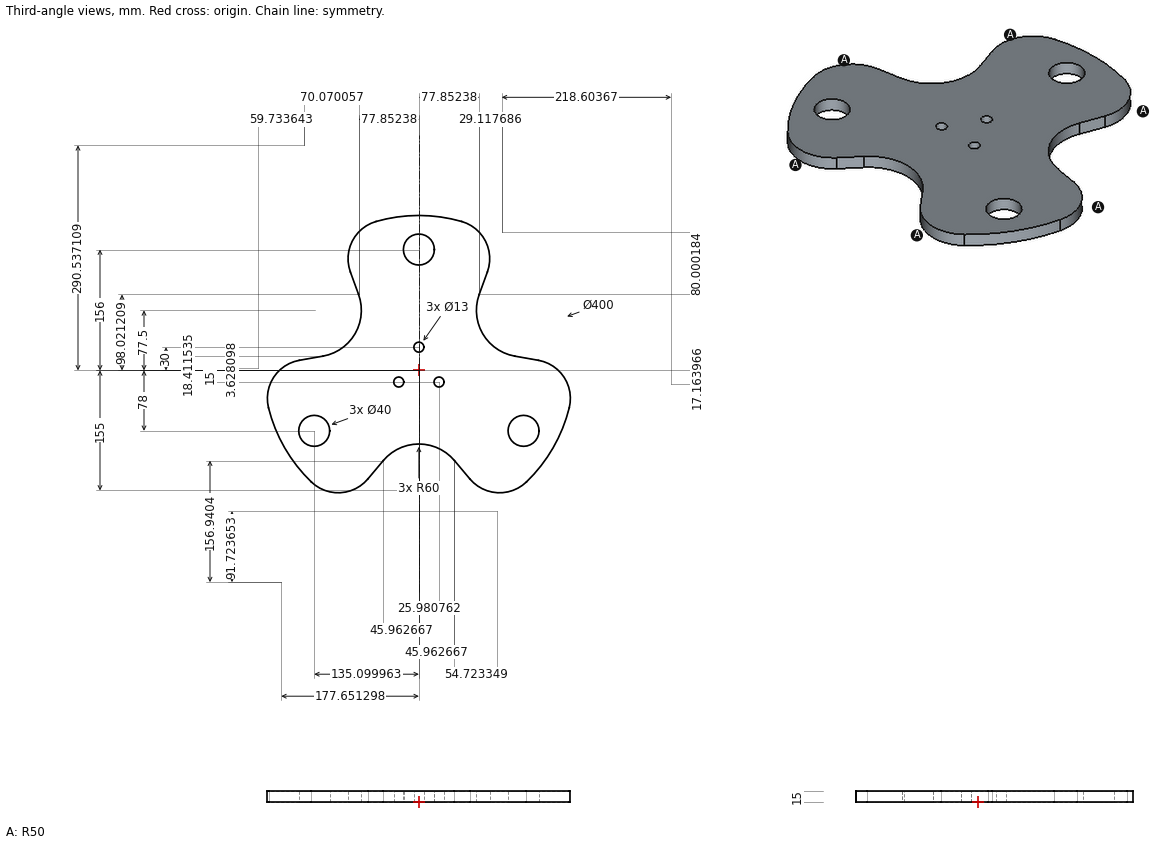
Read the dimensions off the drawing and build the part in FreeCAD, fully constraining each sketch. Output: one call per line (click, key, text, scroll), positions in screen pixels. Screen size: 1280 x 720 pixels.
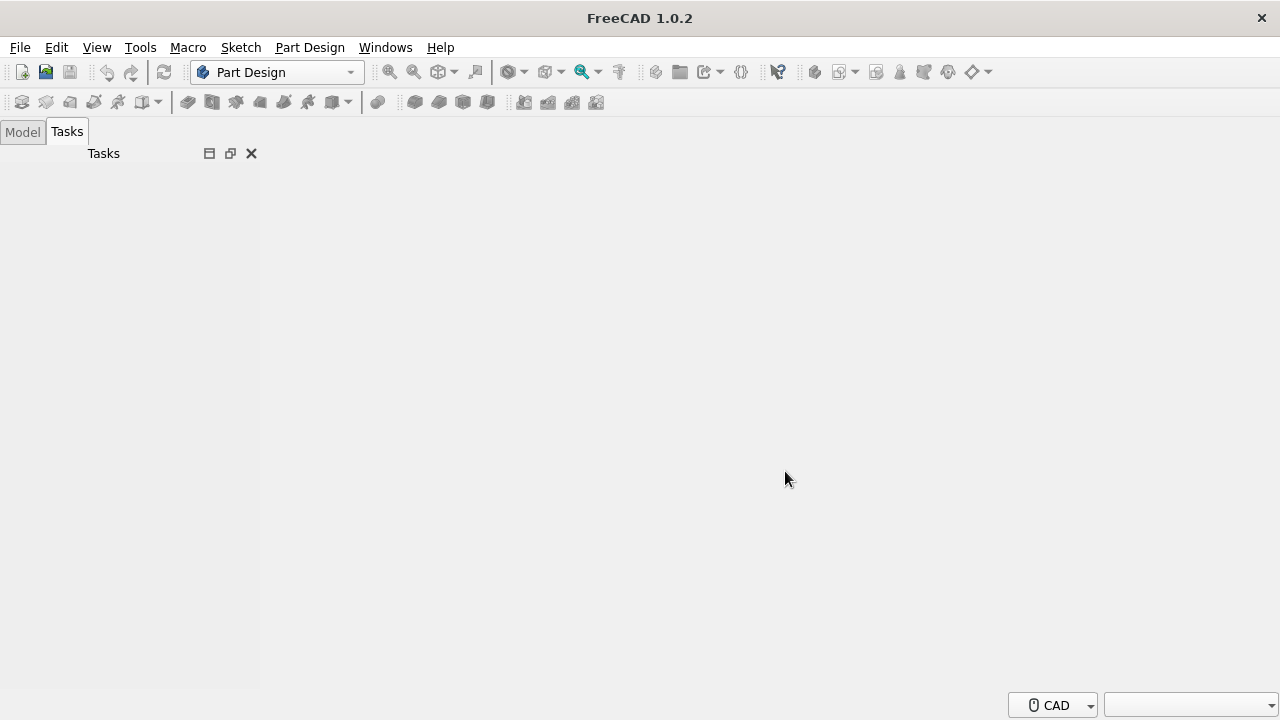
click(22, 72)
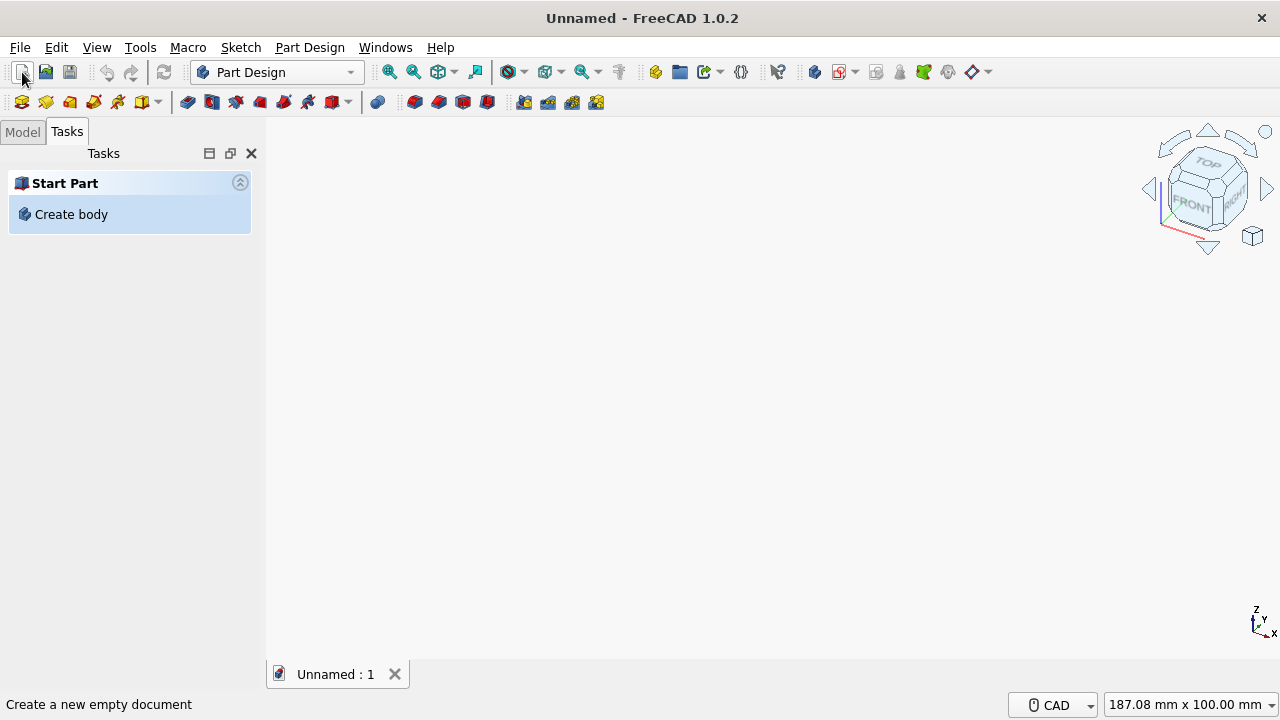
click(840, 72)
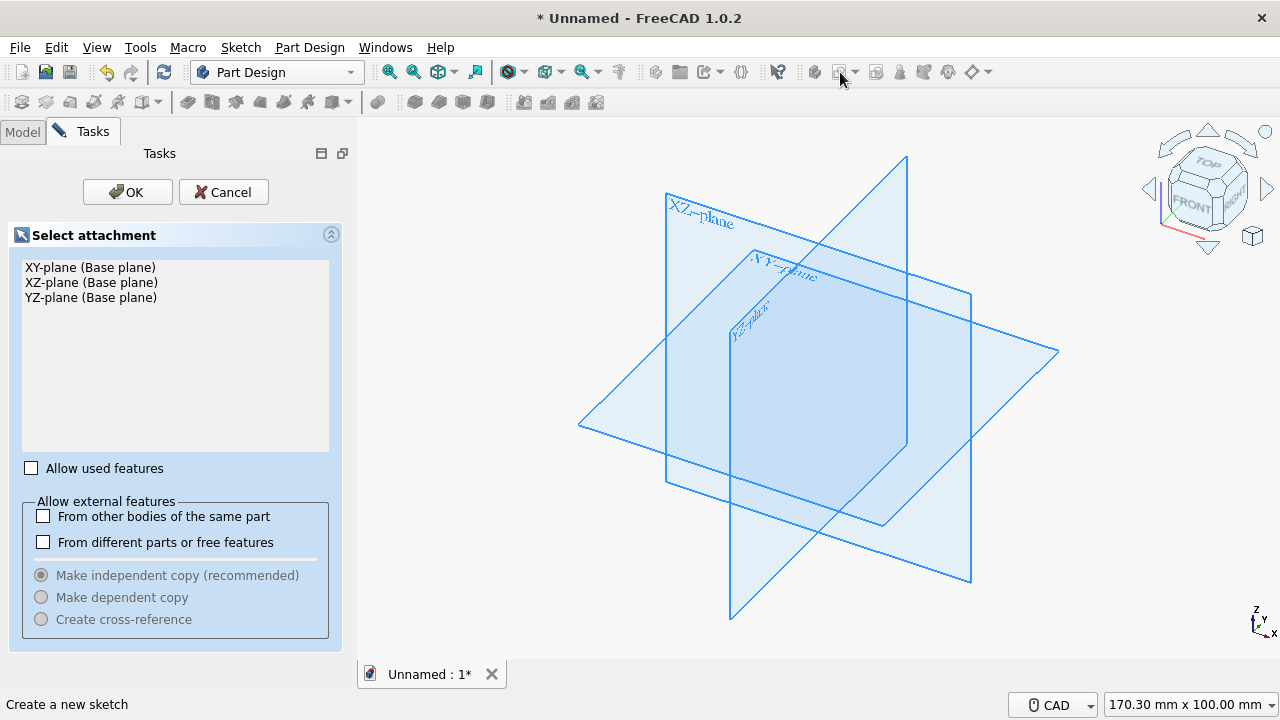
click(82, 268)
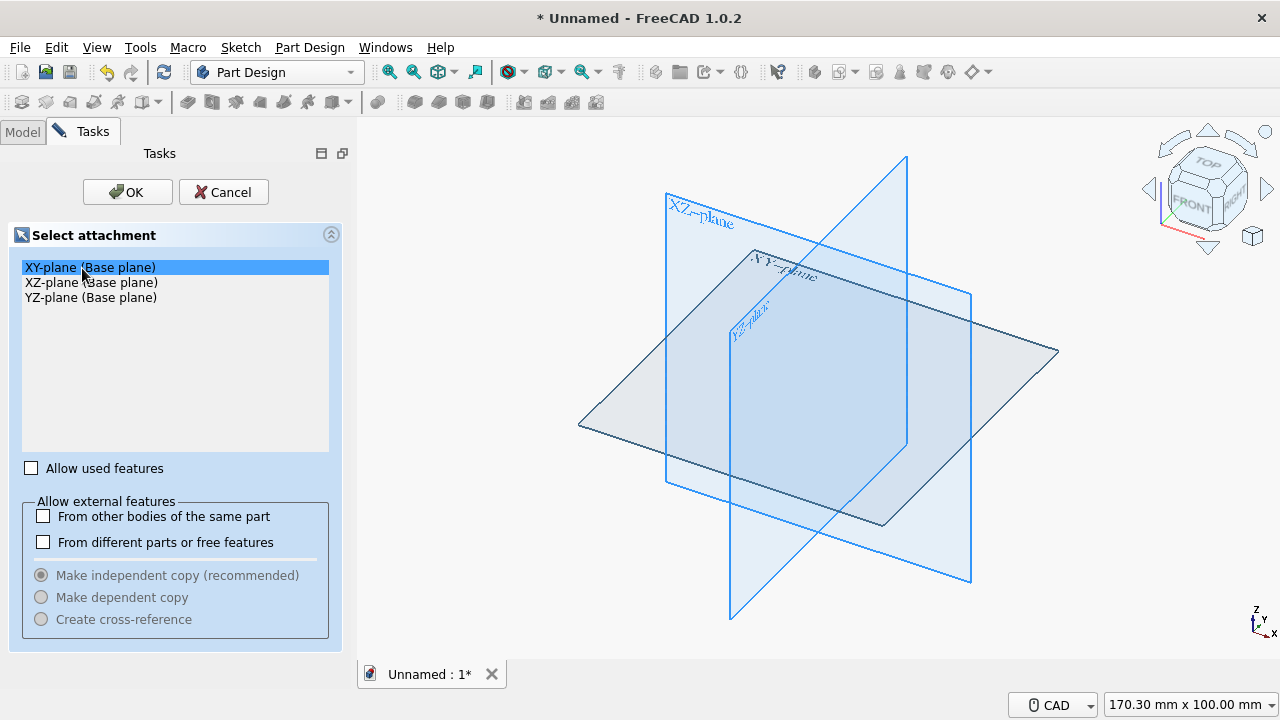
click(128, 192)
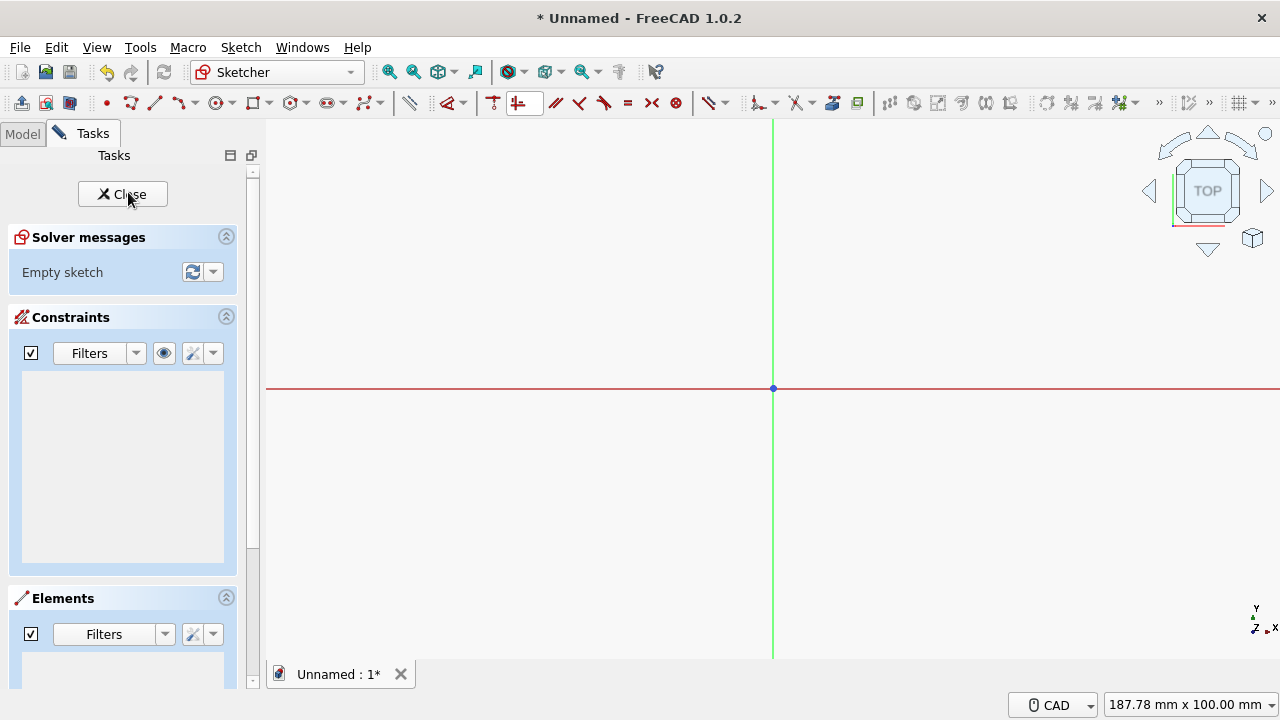
scroll(691, 389, down, 9)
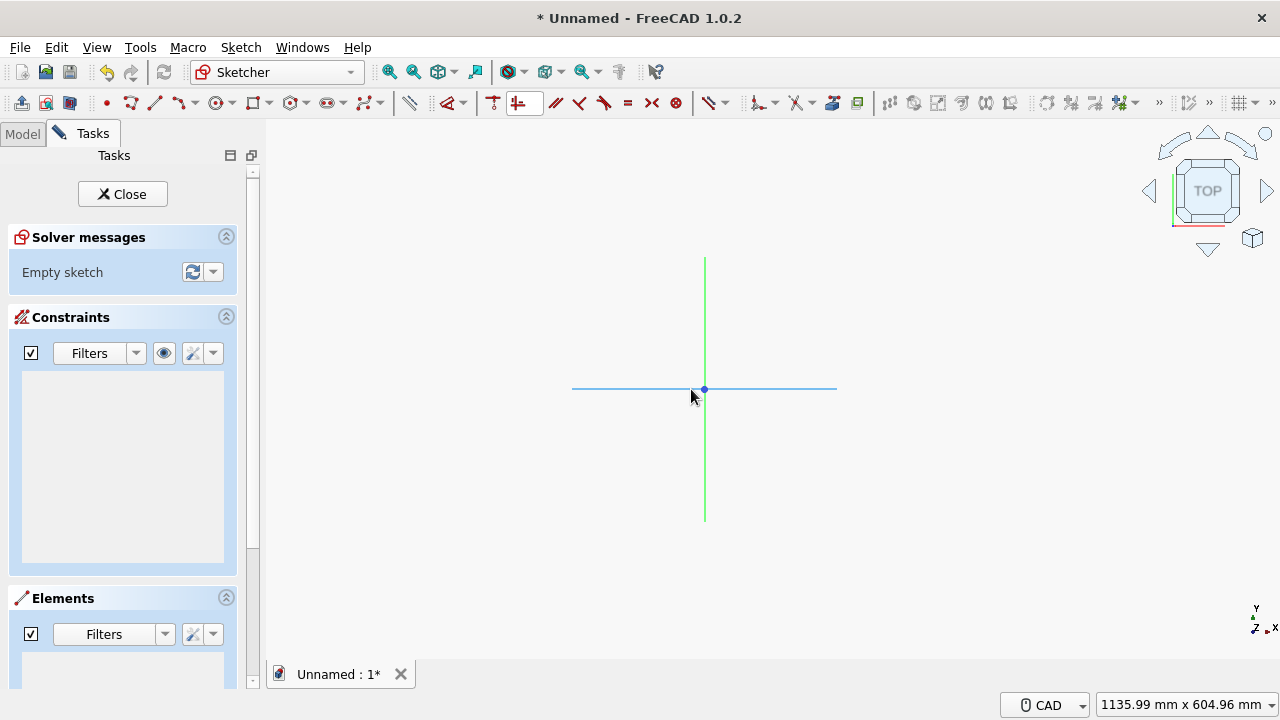
click(216, 104)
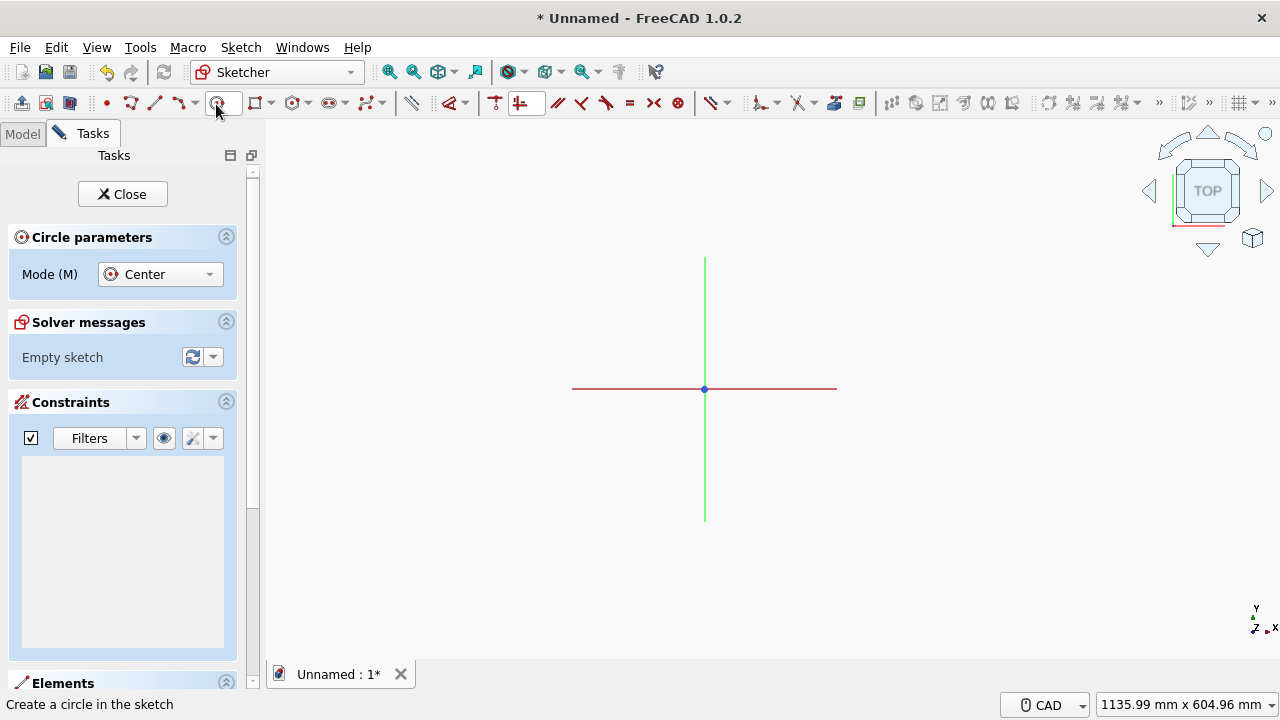
click(705, 389)
move(831, 263)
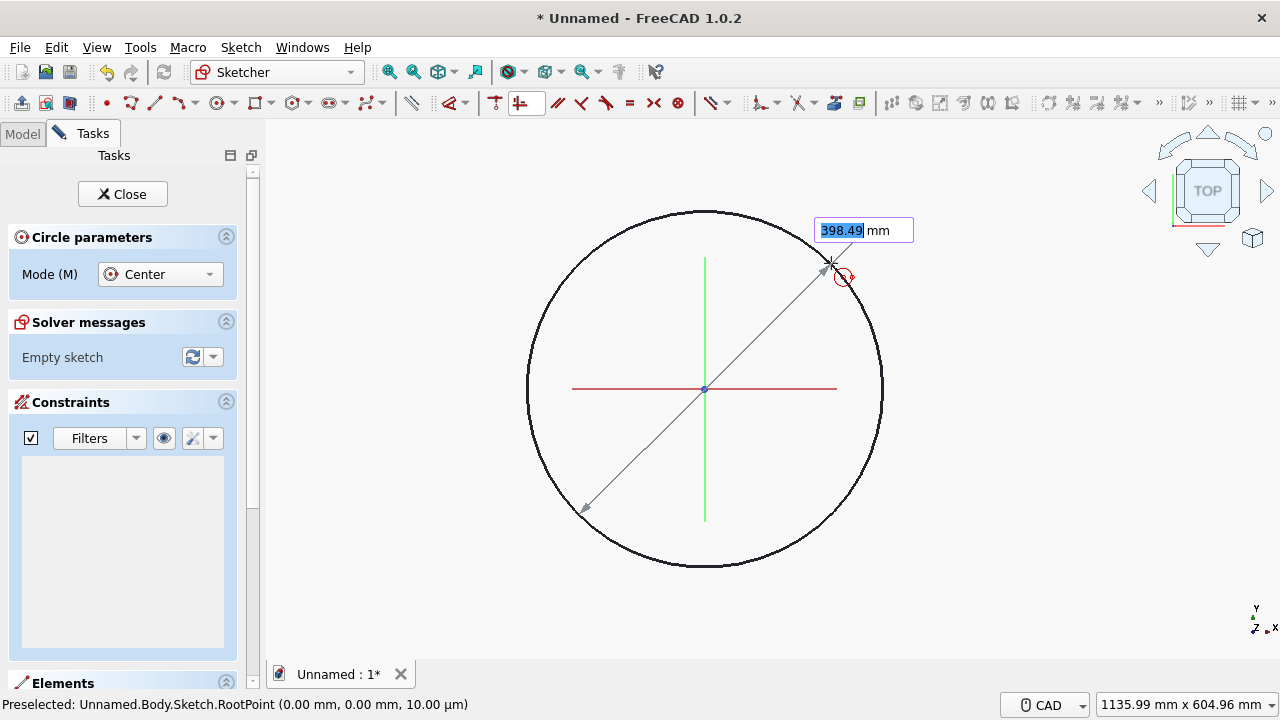
text(400)
key(Return)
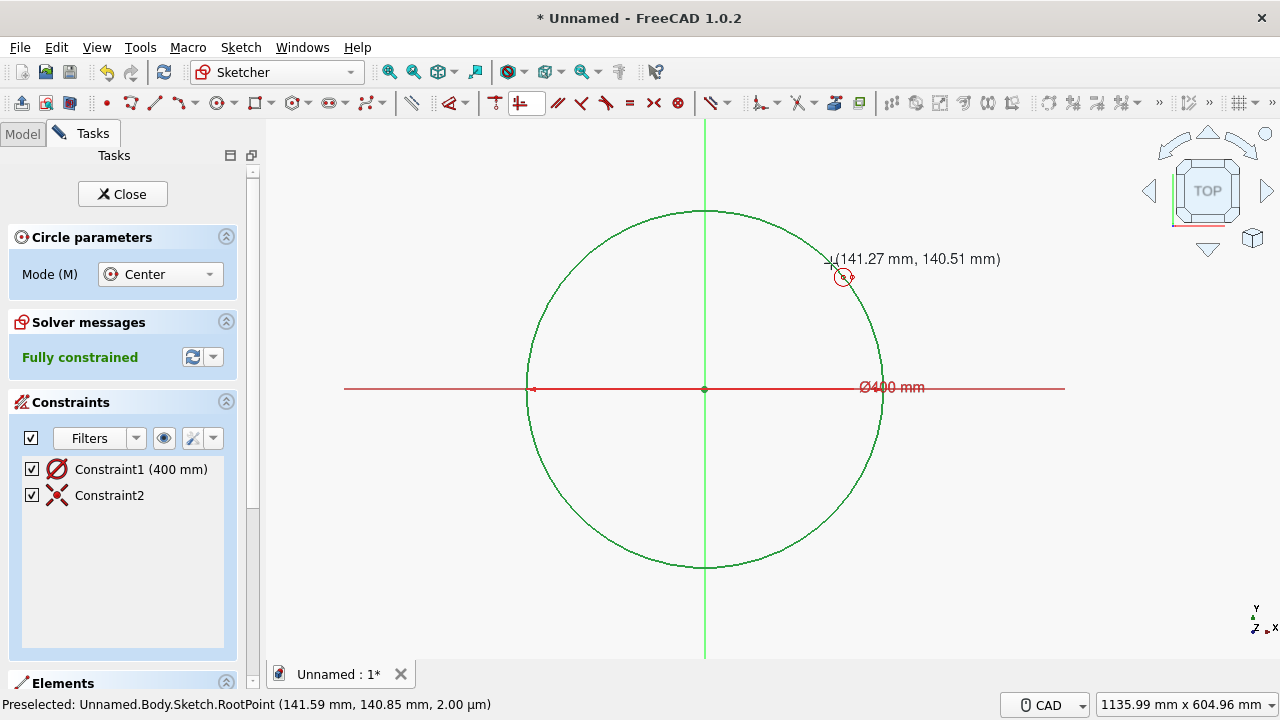
scroll(584, 459, up, 2)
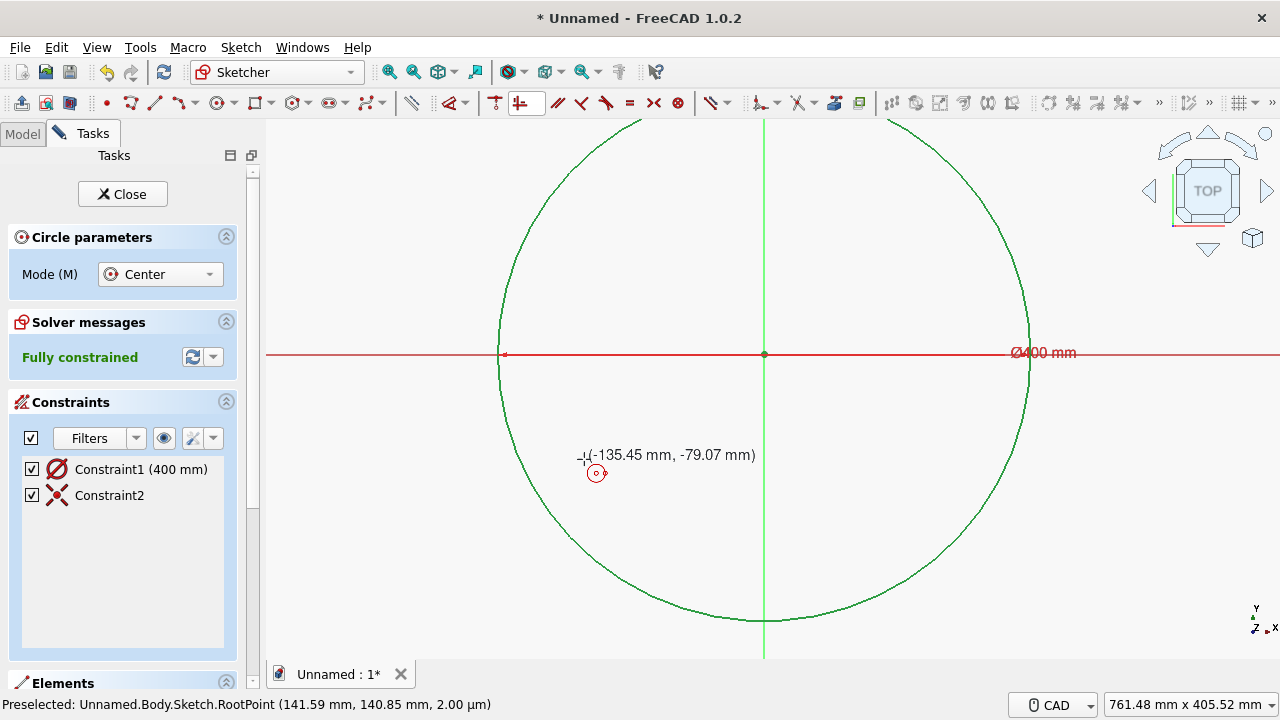
click(584, 459)
move(603, 440)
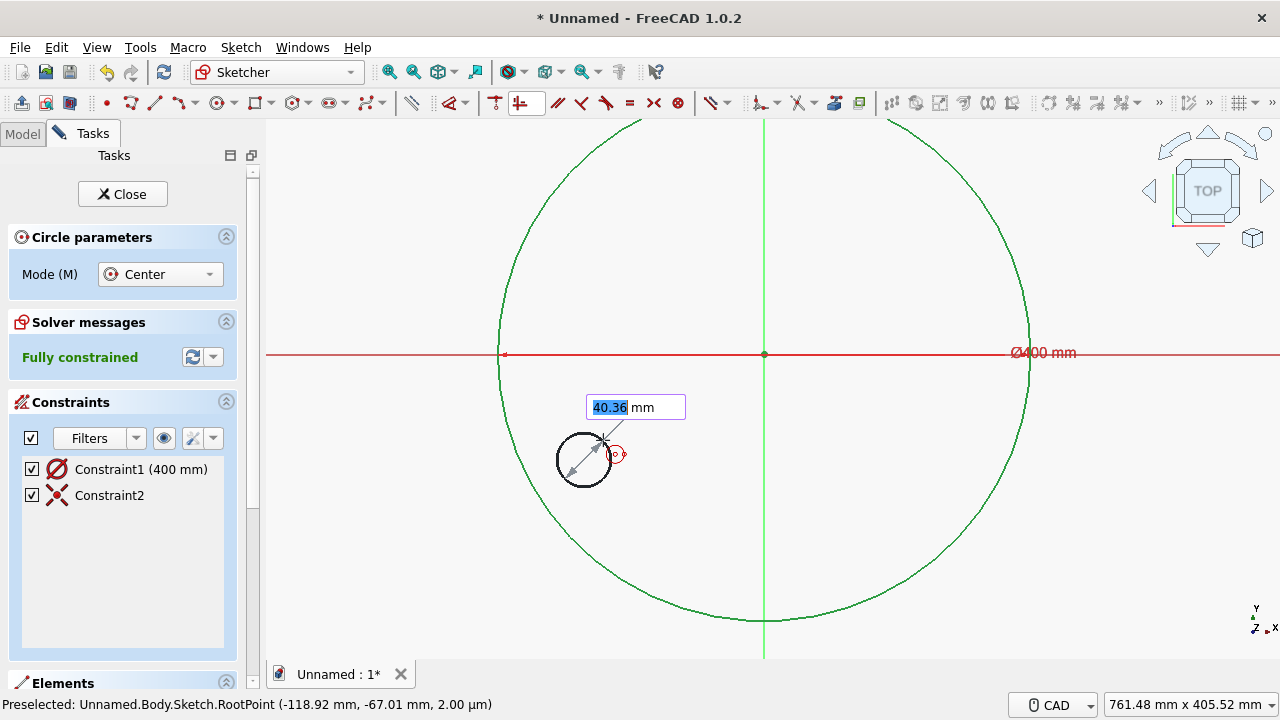
text(40)
key(Return)